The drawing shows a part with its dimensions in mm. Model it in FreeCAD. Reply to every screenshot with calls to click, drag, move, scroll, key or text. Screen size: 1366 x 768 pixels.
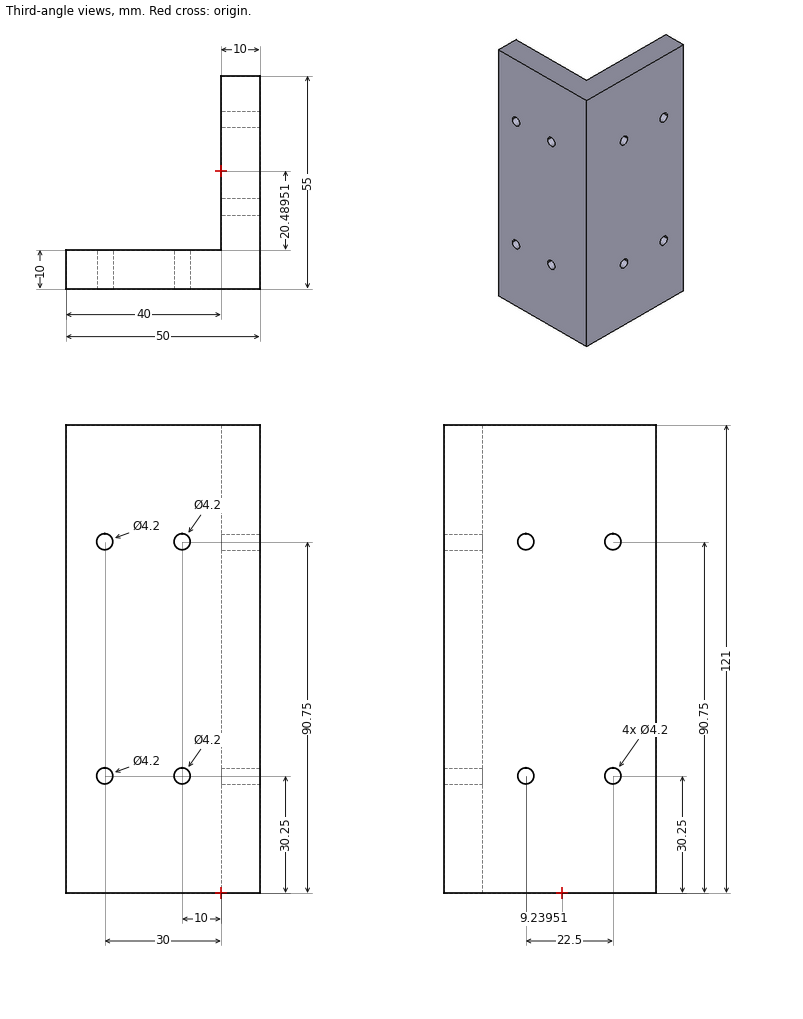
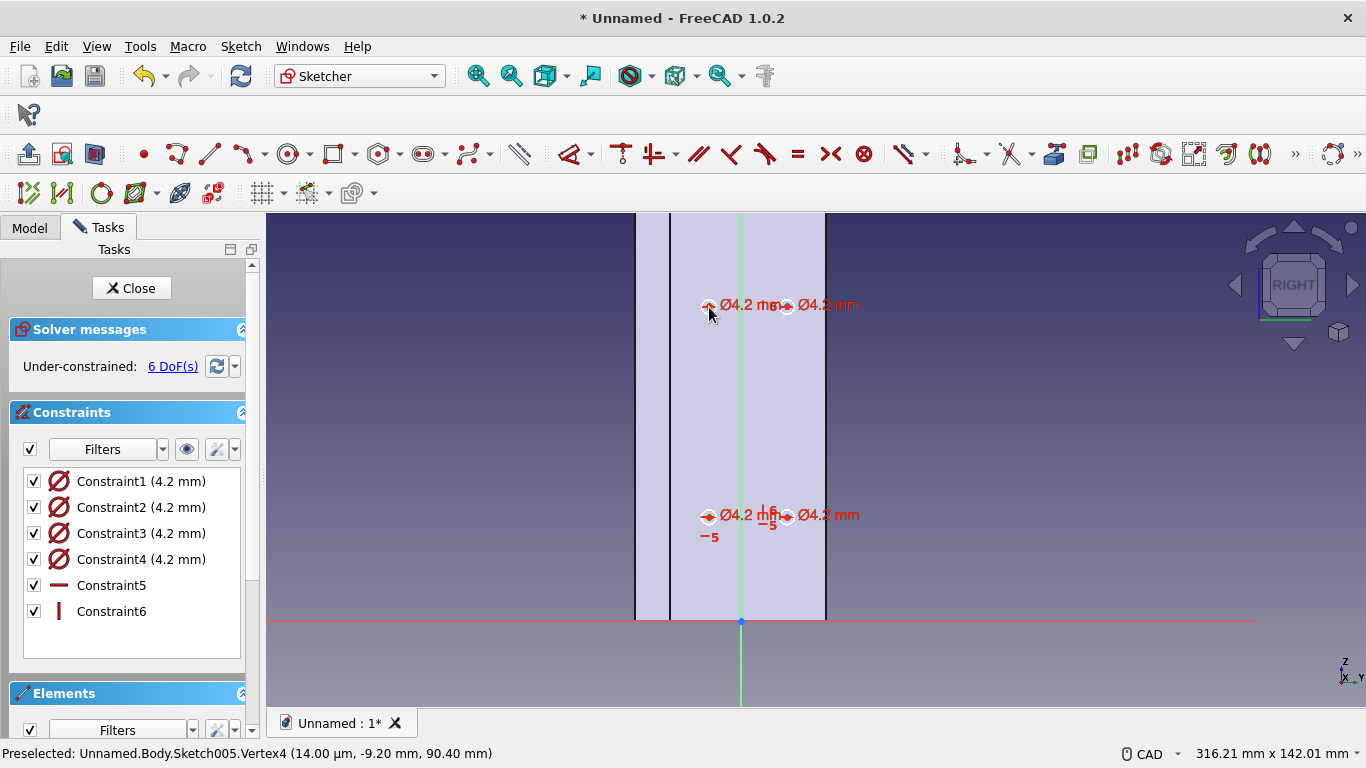
key(v)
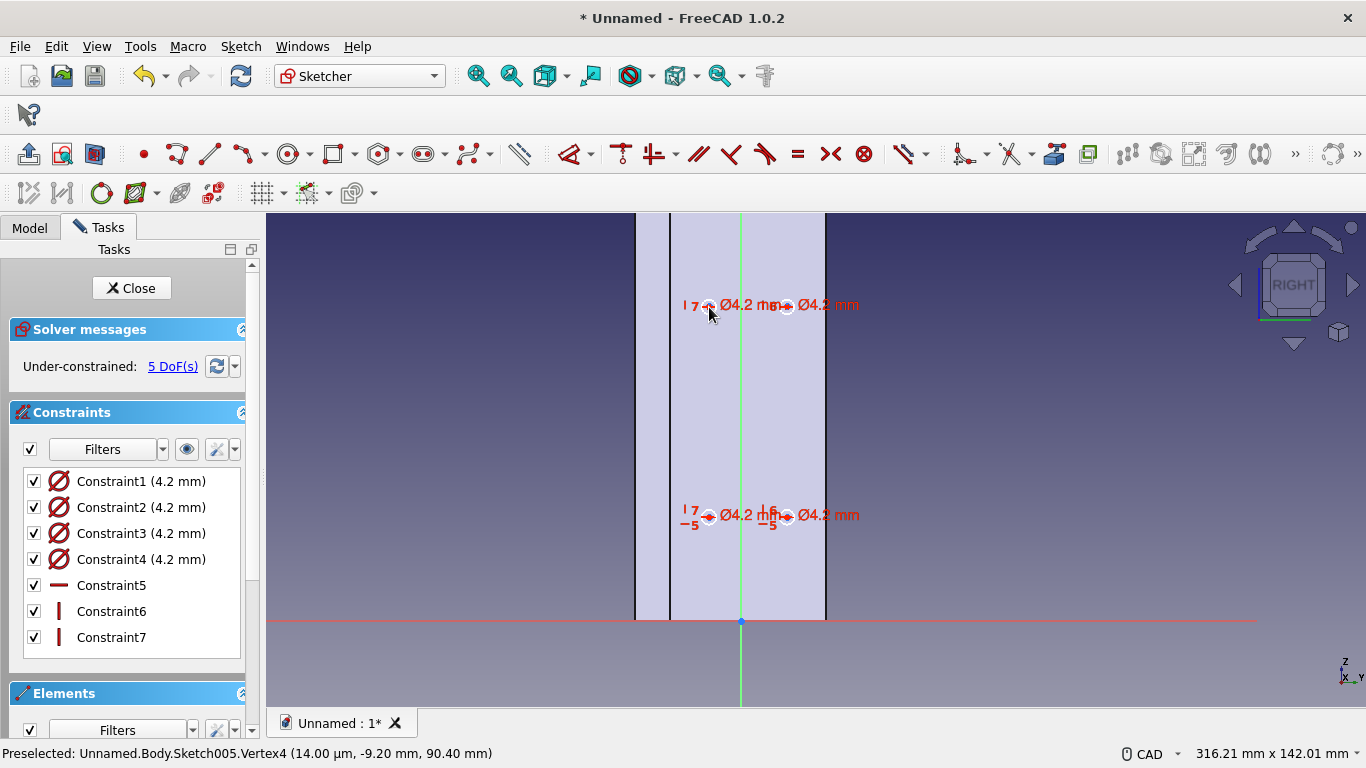
click(787, 307)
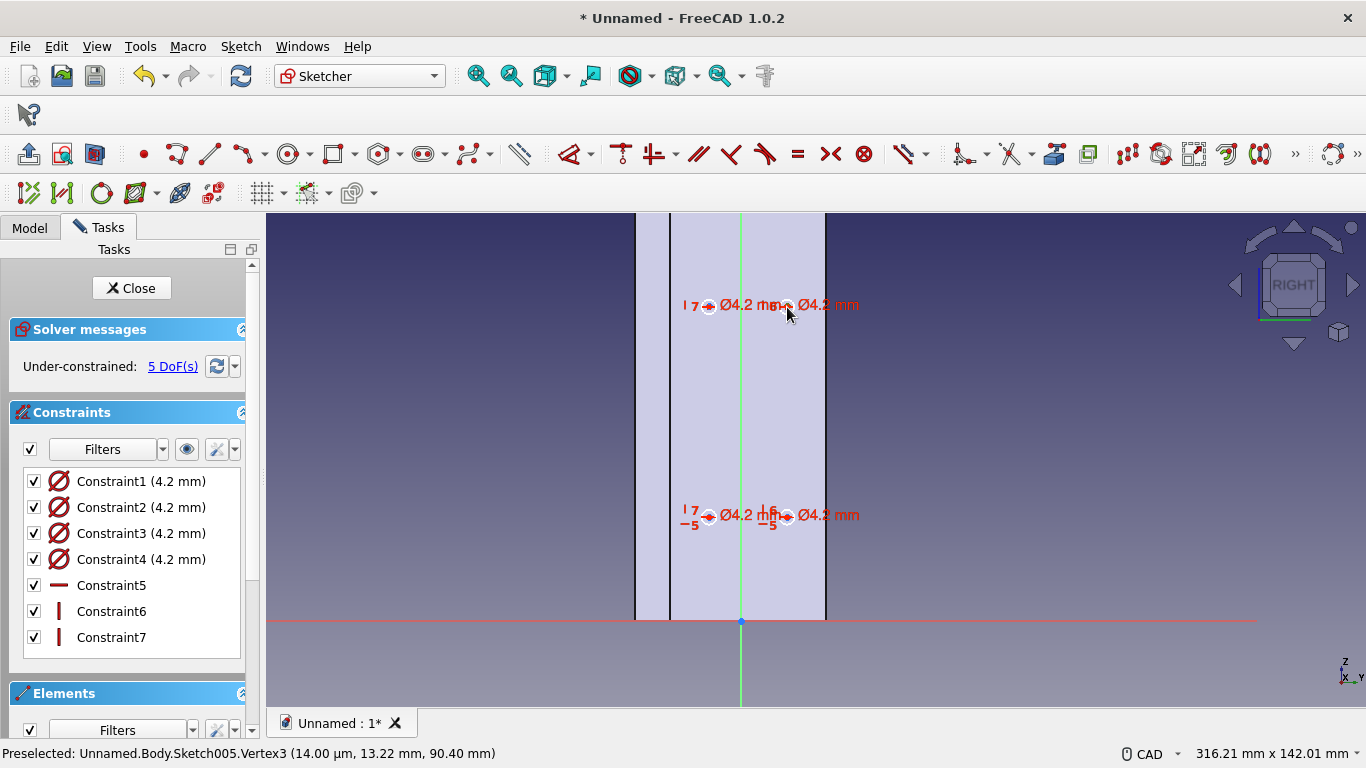
click(709, 307)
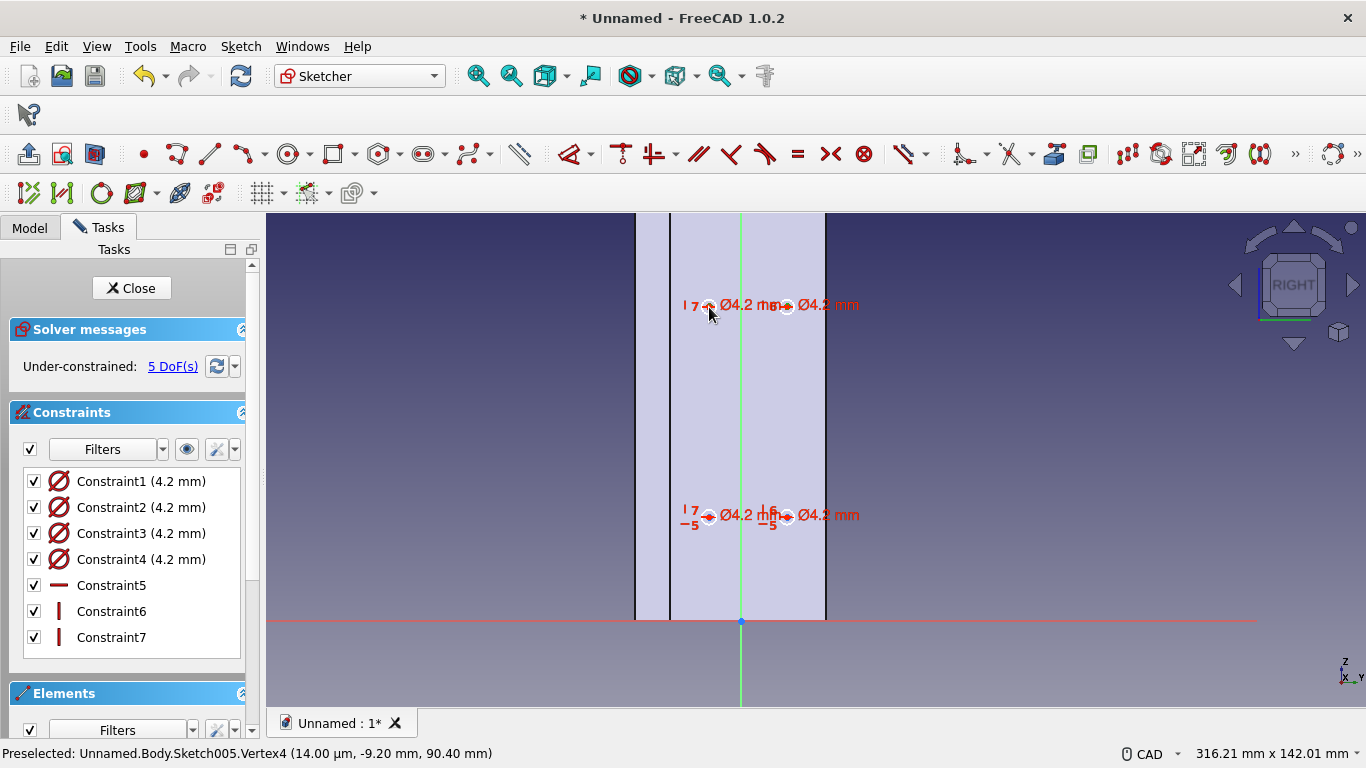
click(676, 154)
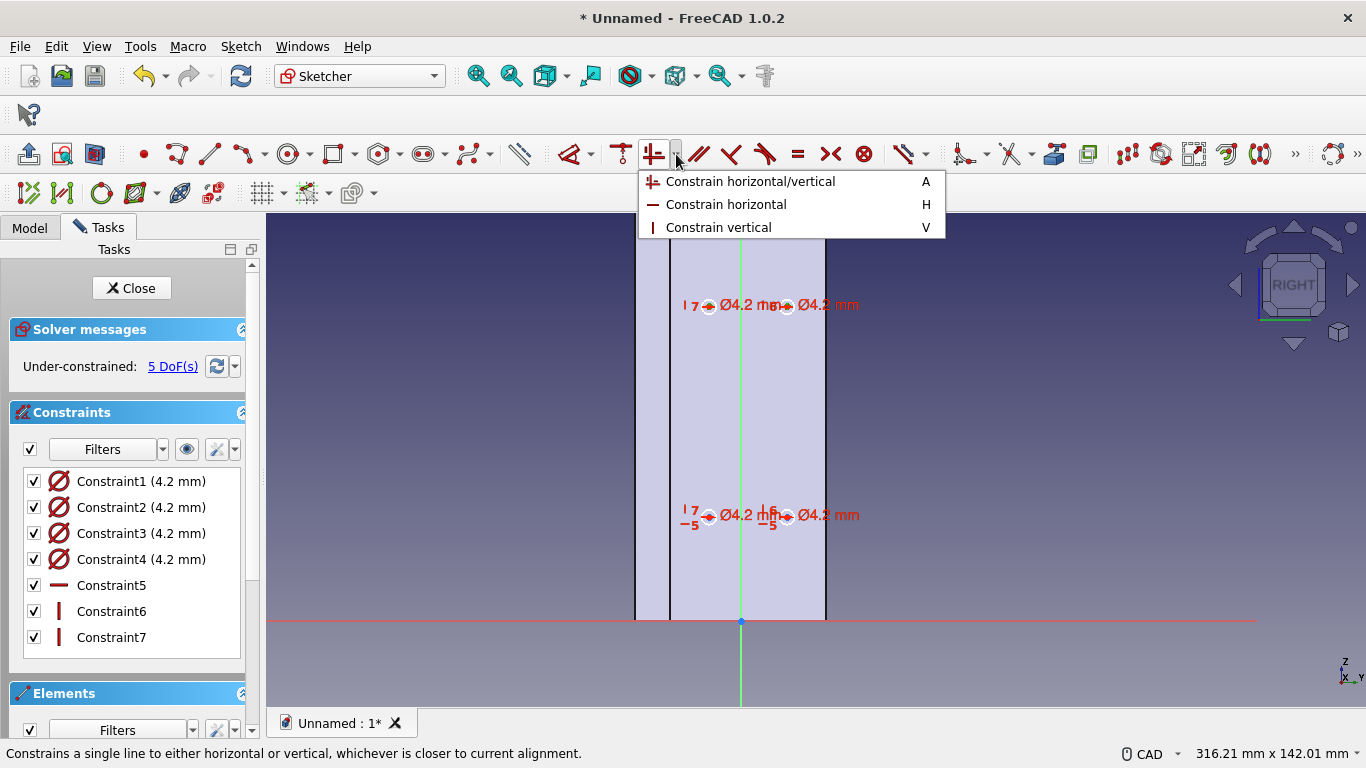
click(792, 204)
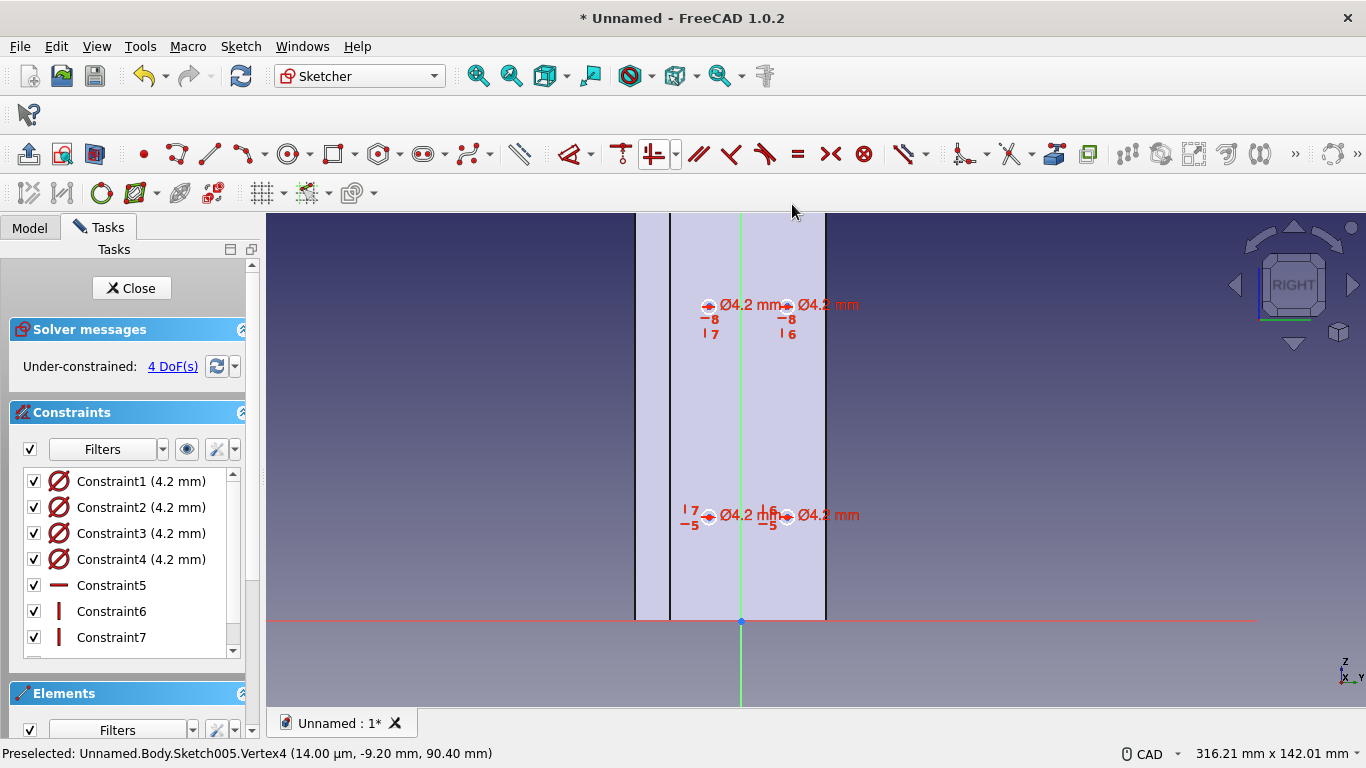
key(d)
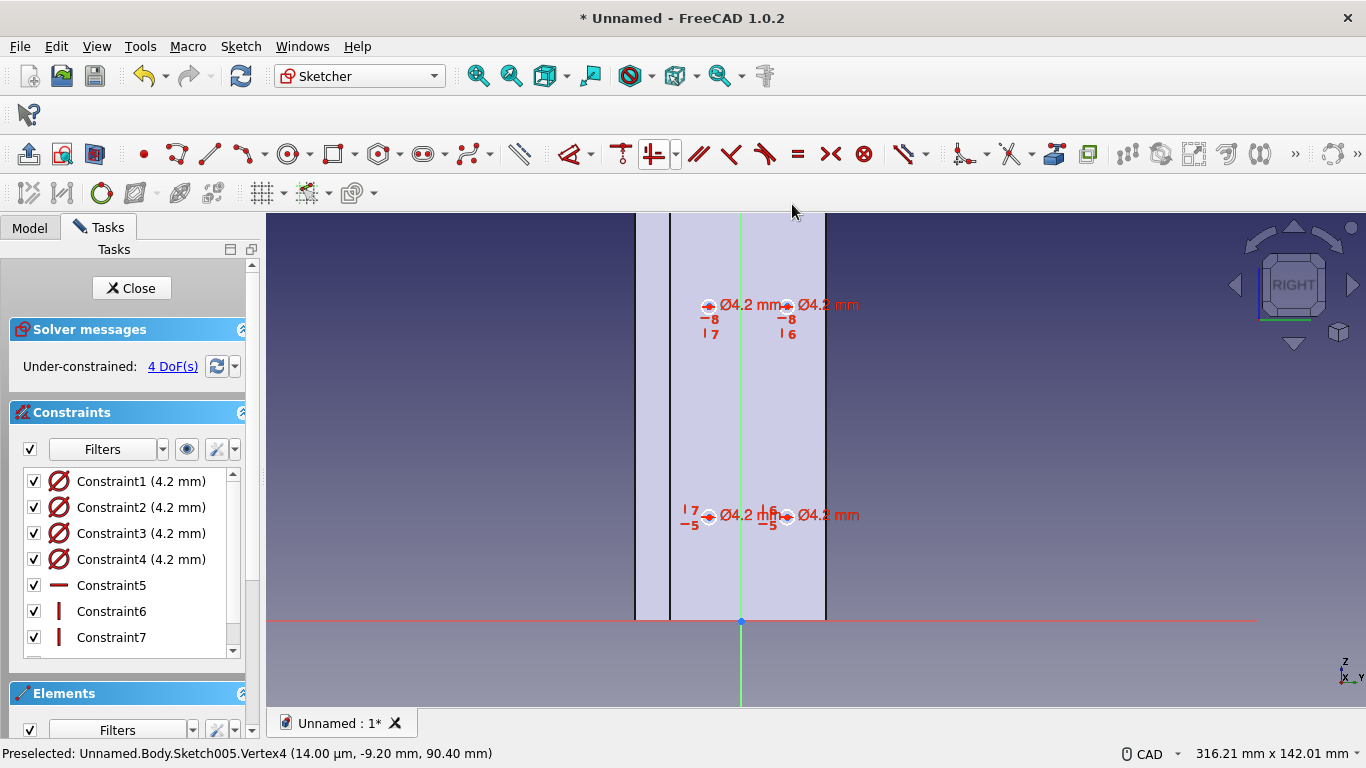
click(787, 517)
click(821, 569)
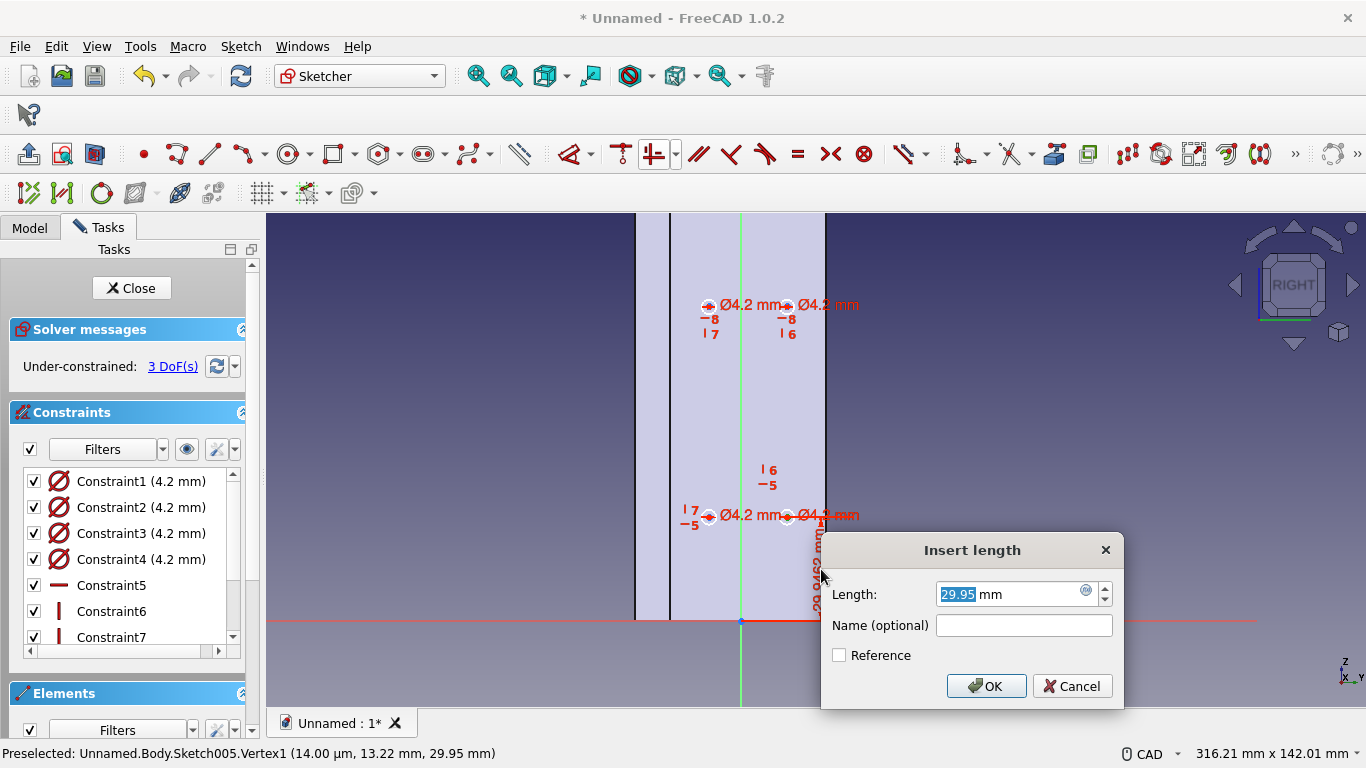
text(30.25)
key(Return)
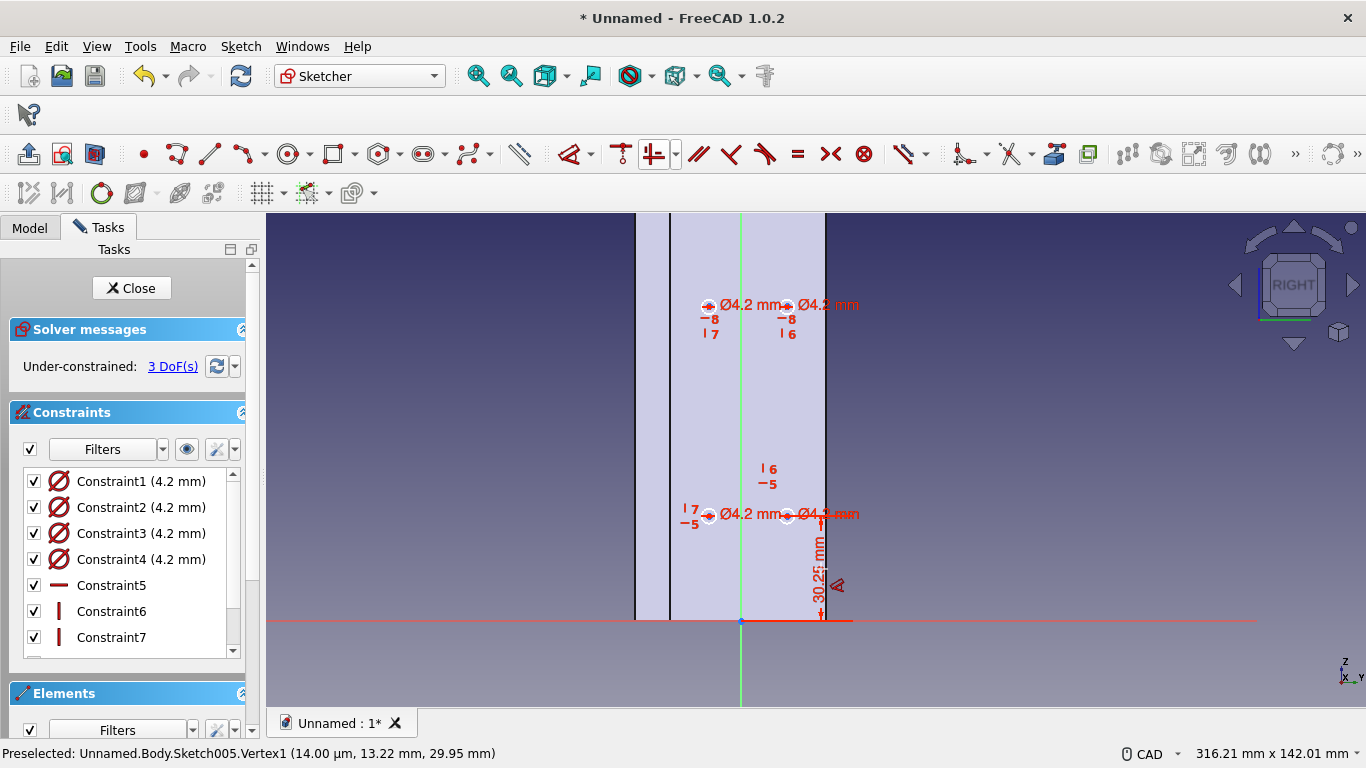
click(787, 307)
click(821, 464)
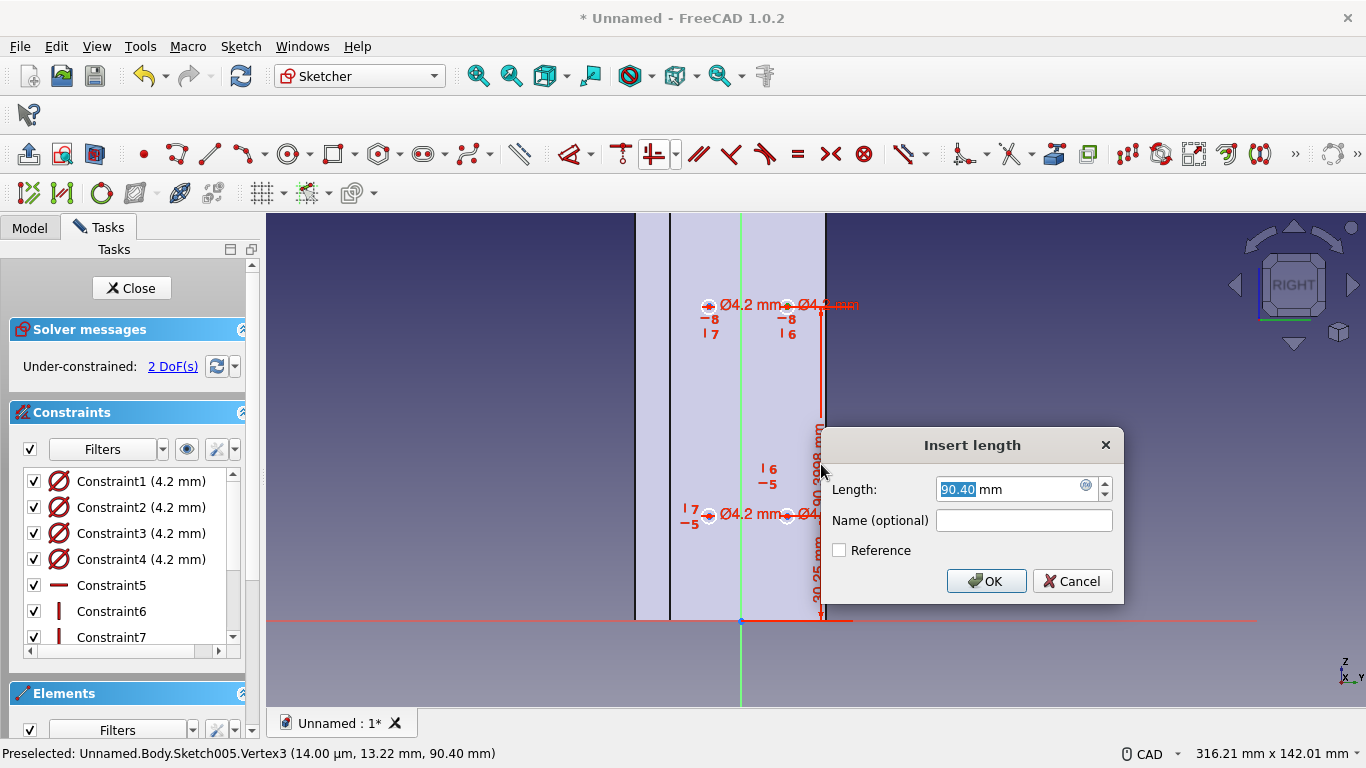
text(90.75)
key(Return)